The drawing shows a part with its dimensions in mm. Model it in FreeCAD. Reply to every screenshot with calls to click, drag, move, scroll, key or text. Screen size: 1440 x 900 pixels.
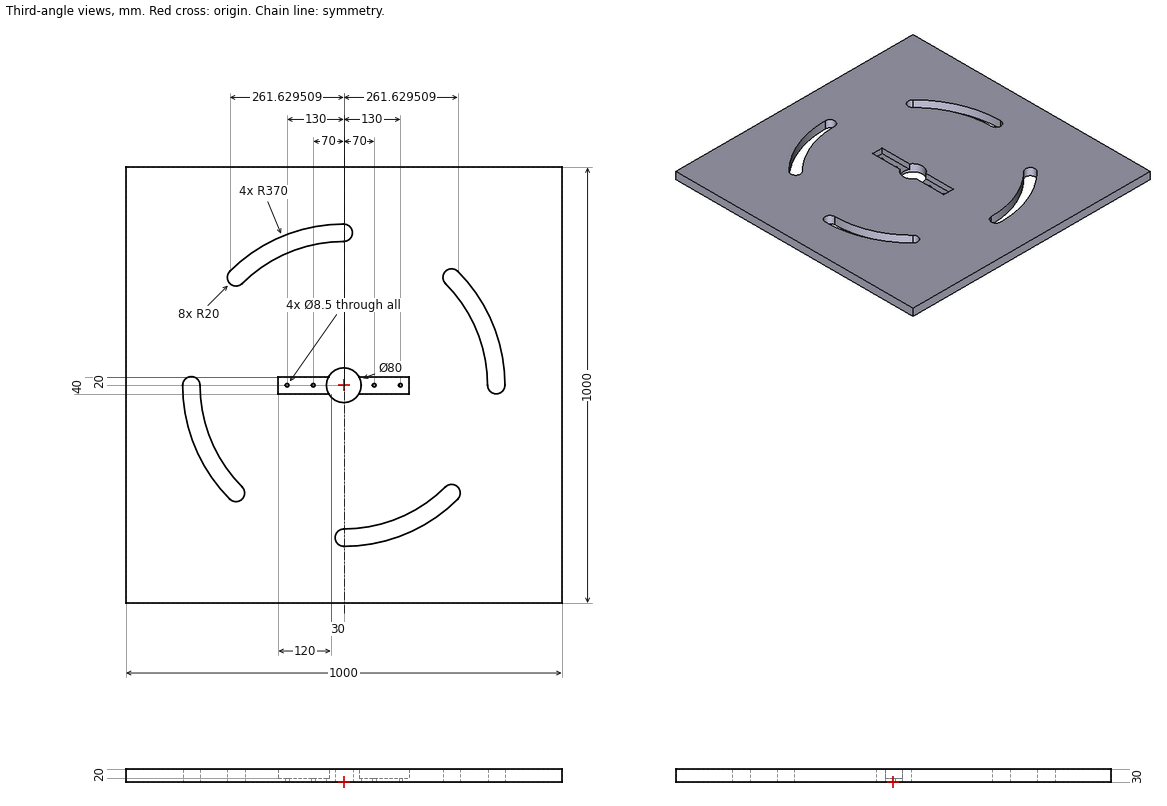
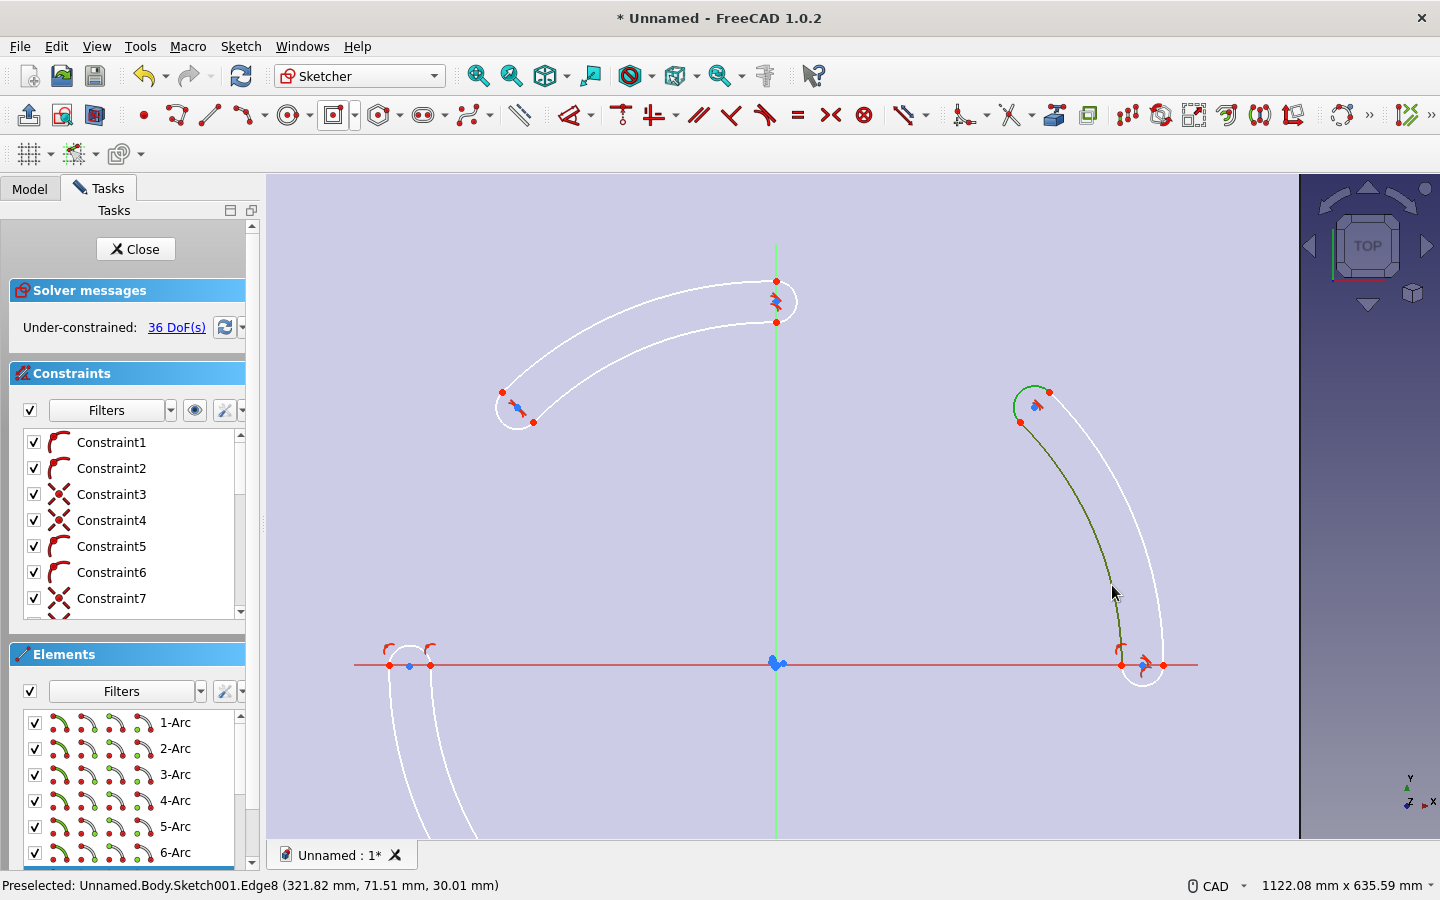
key(t)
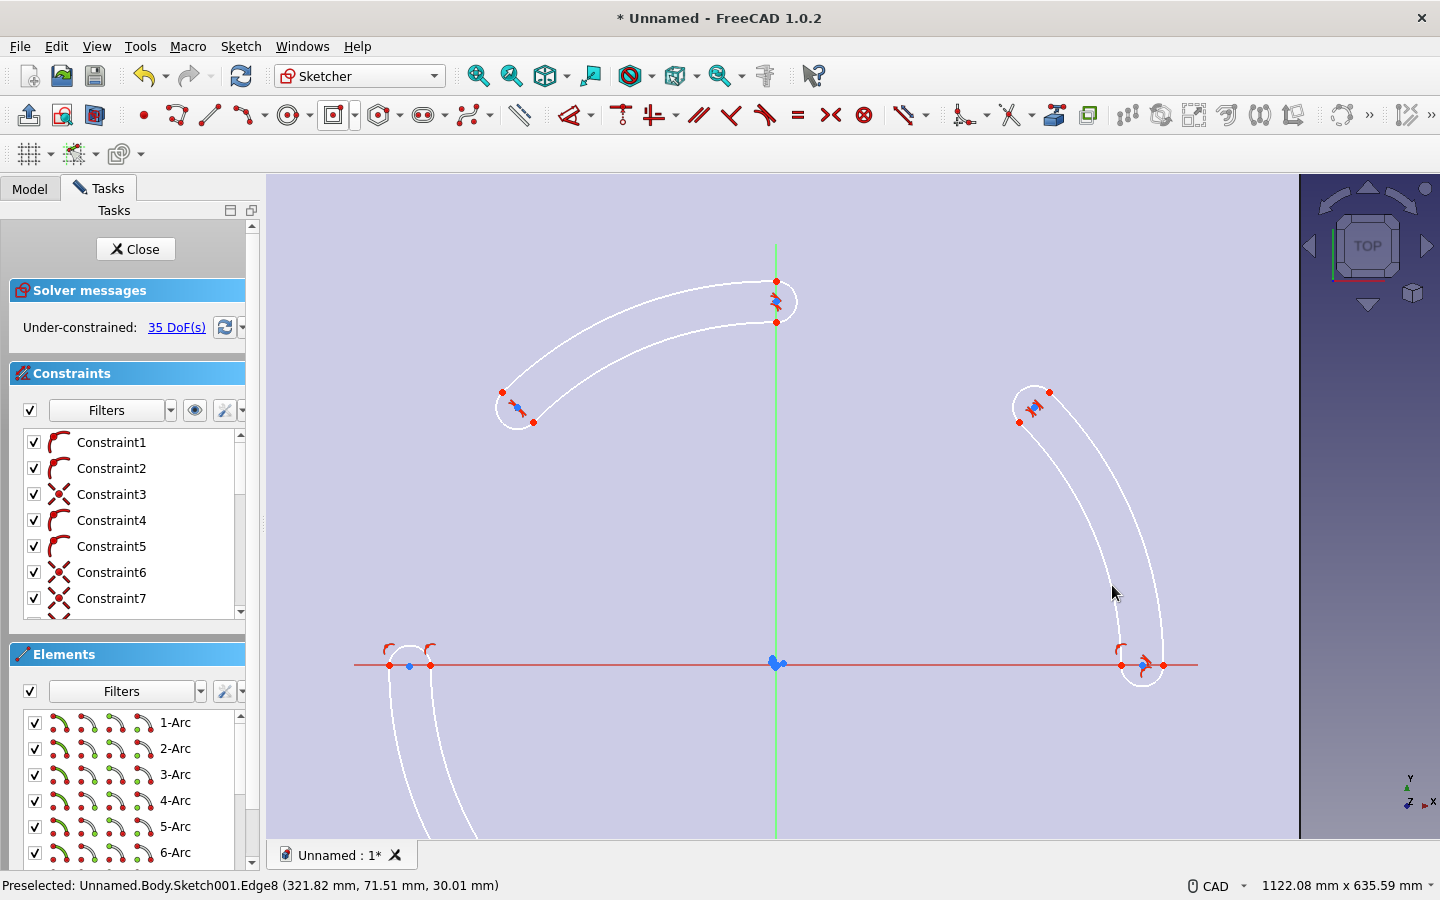
scroll(794, 313, down, 3)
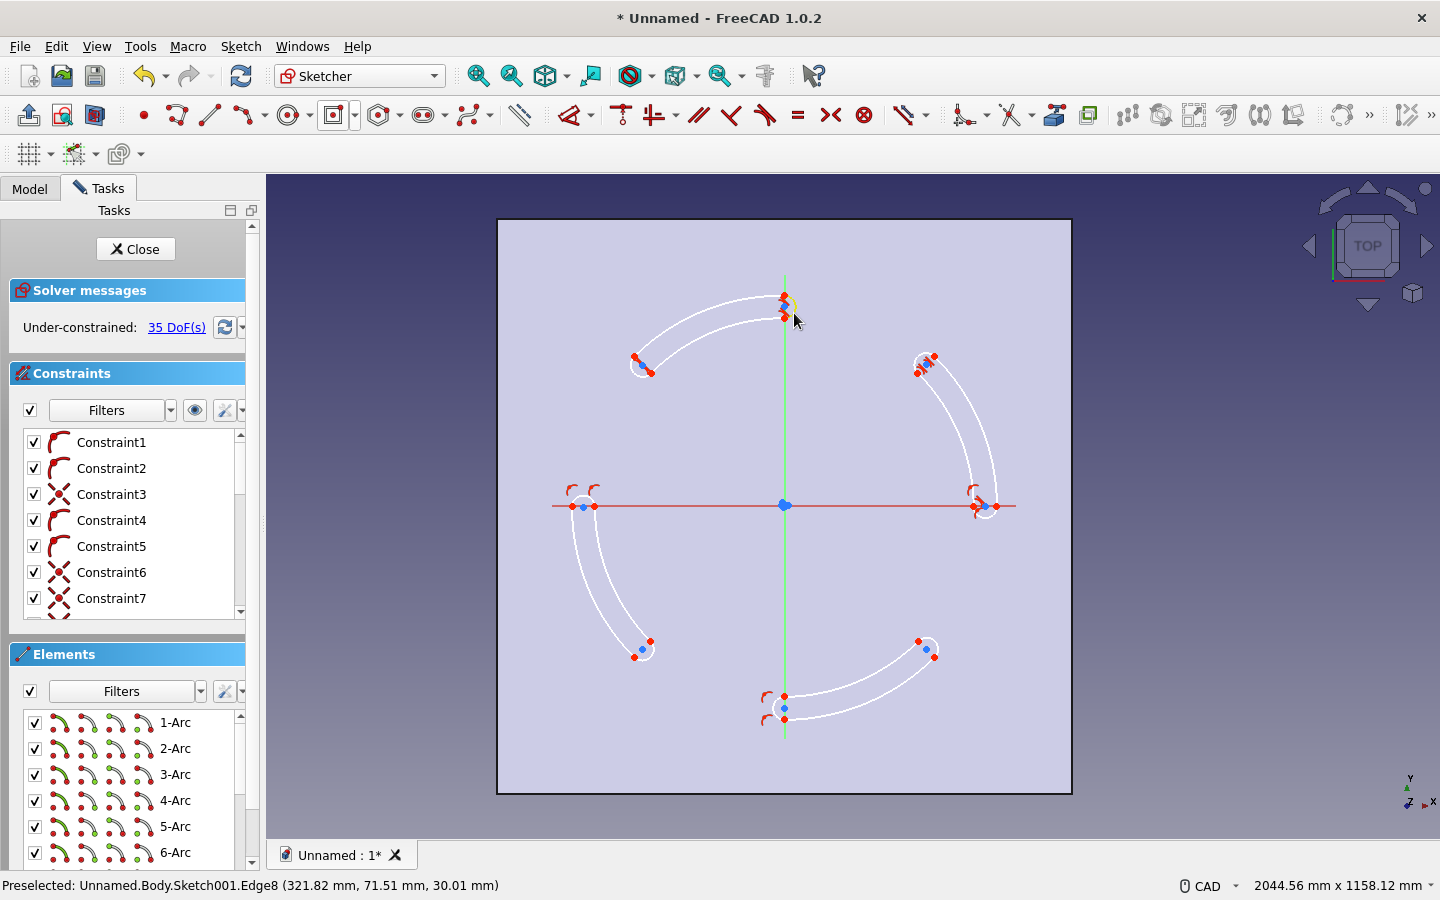
scroll(775, 702, up, 3)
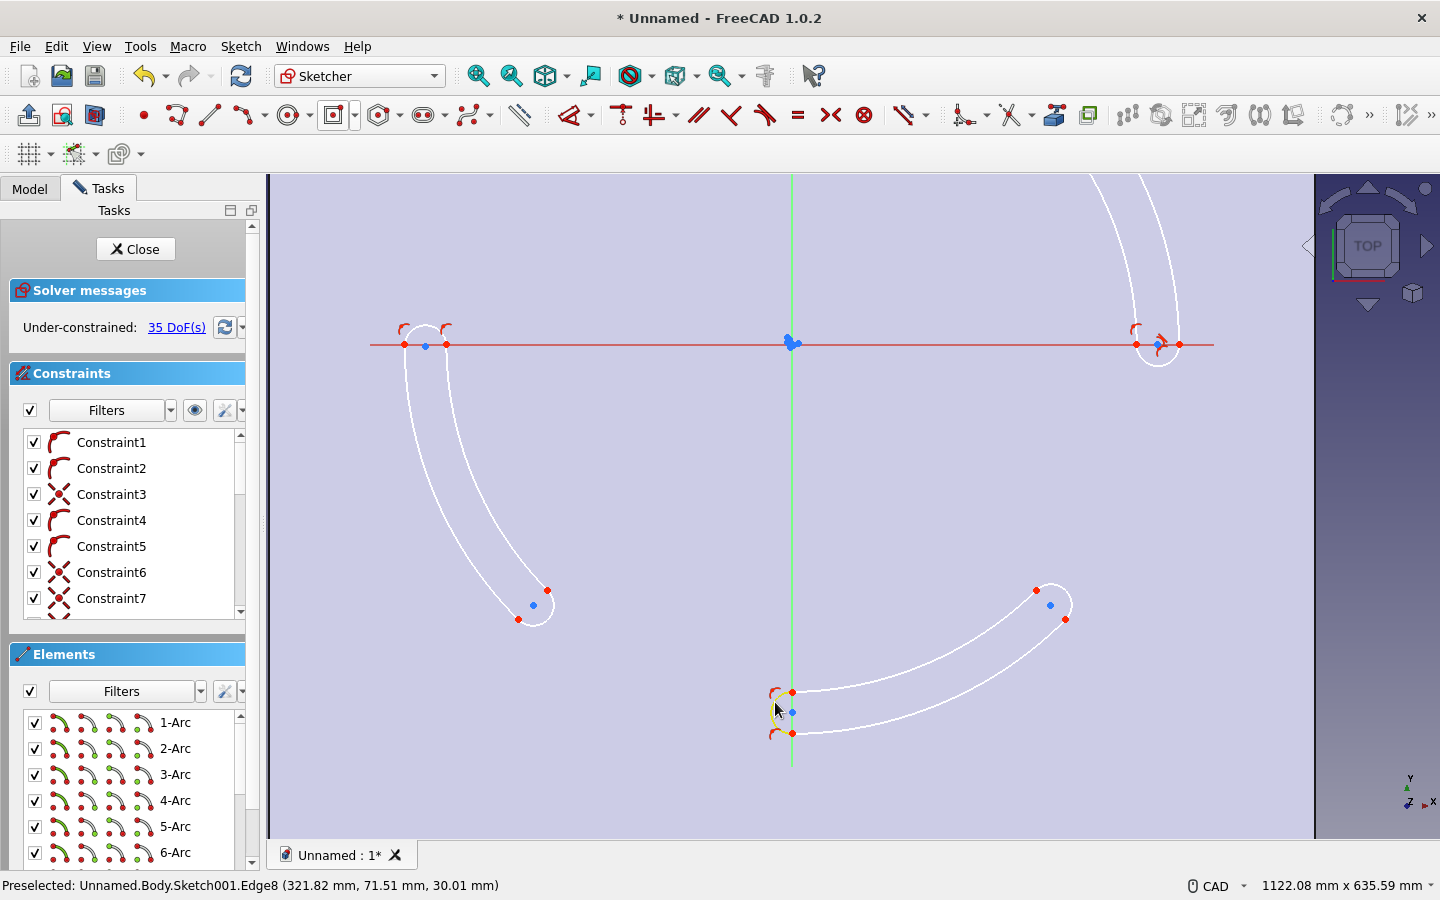
click(775, 701)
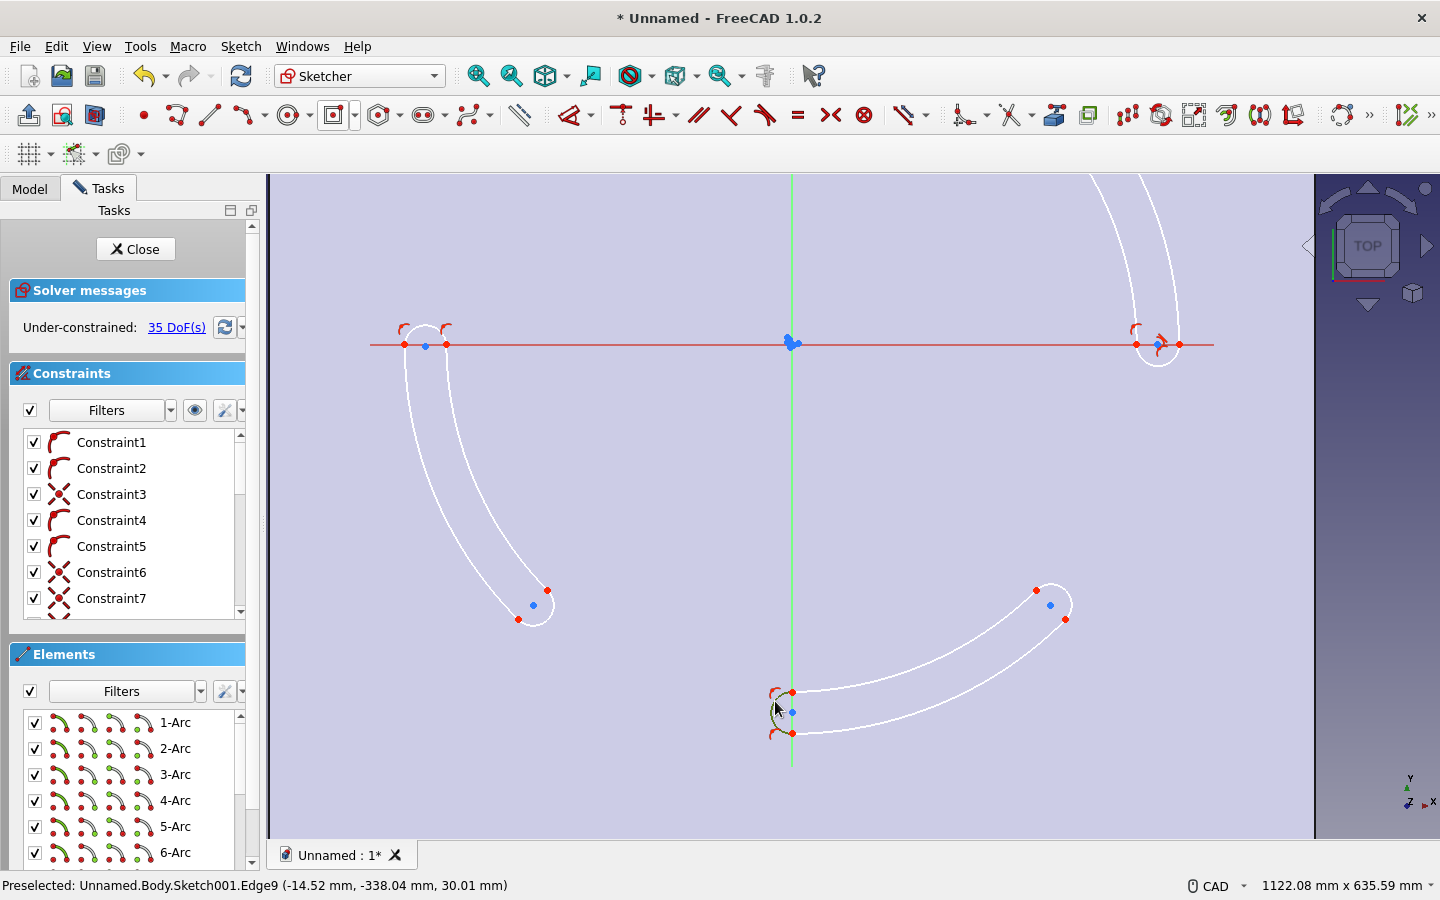
click(882, 723)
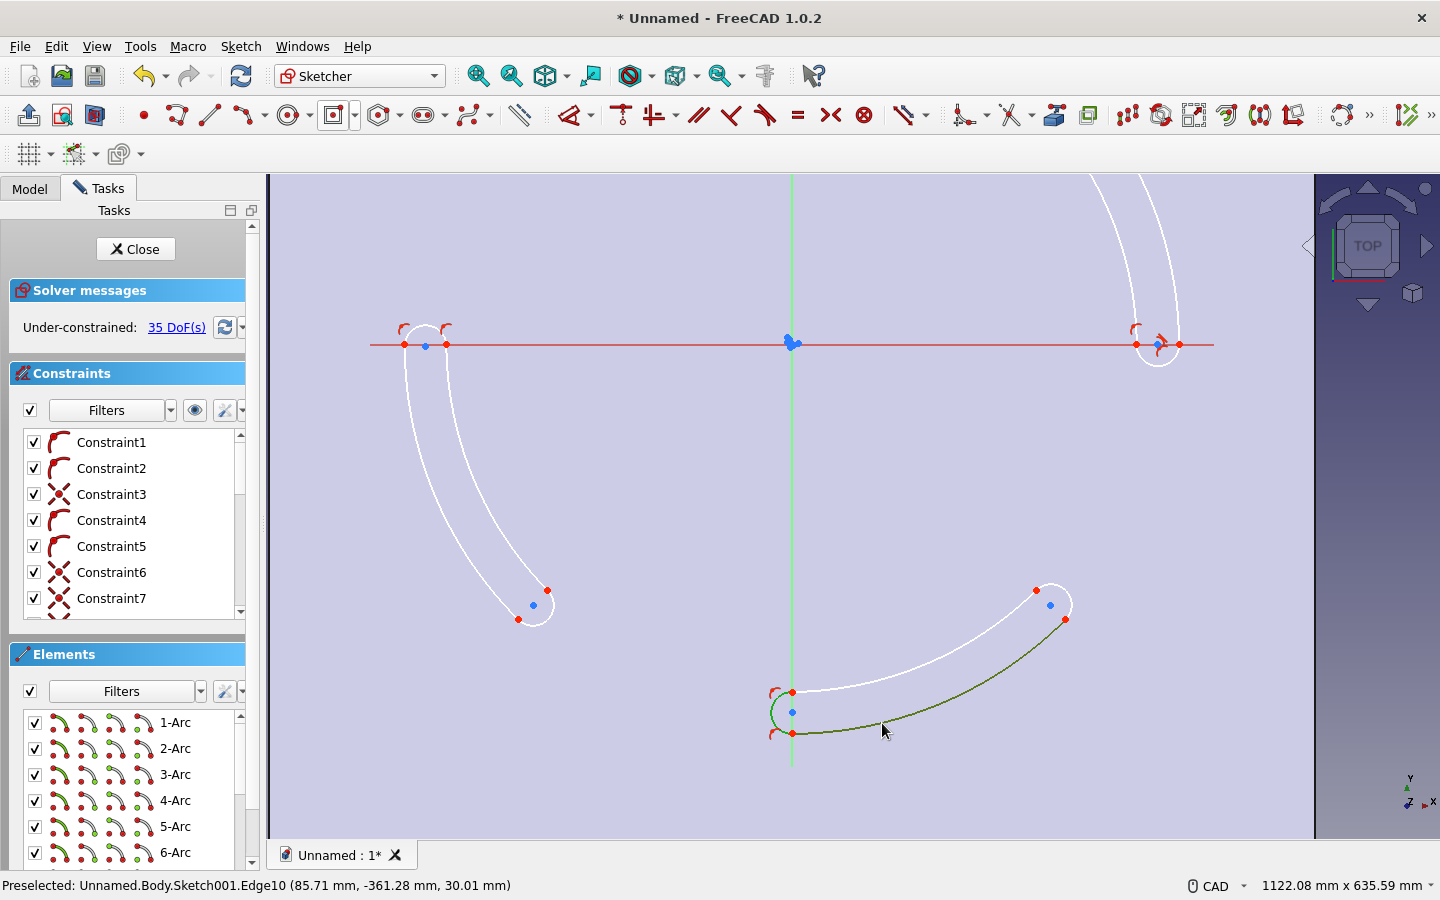
click(765, 116)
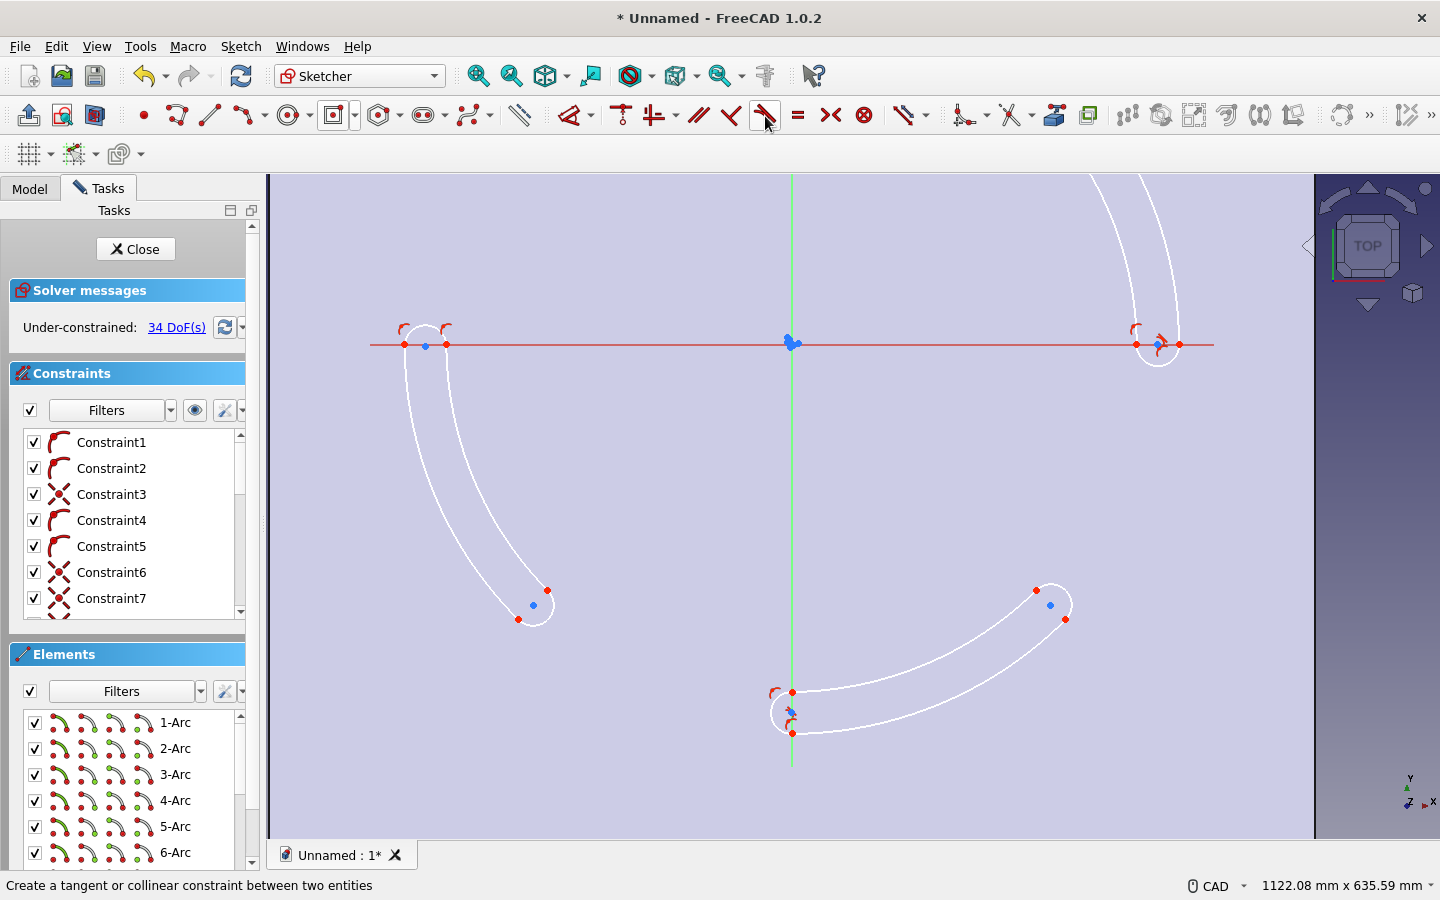
click(882, 723)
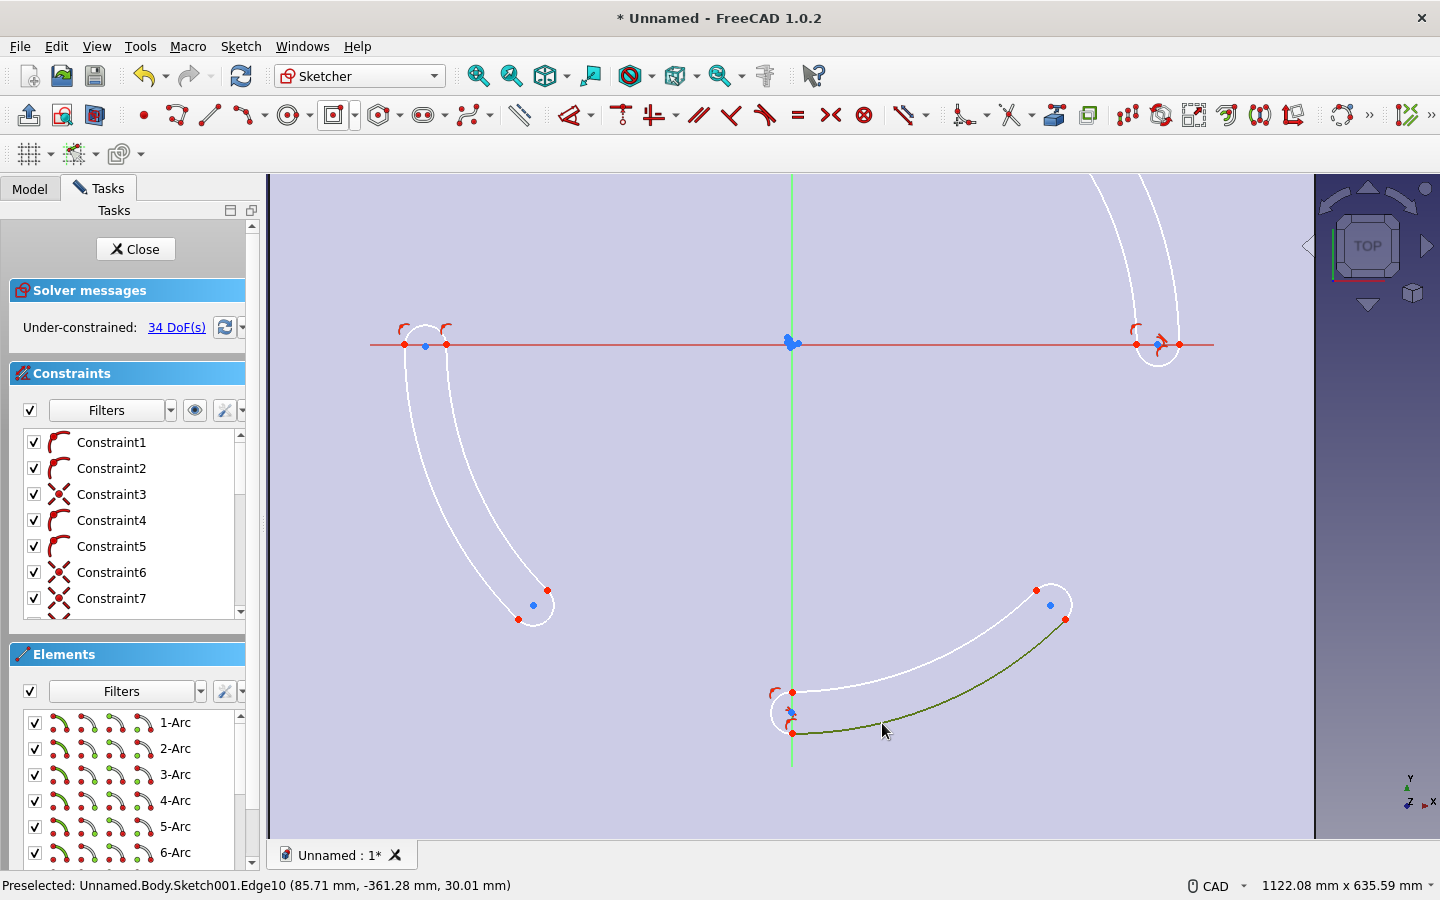
click(1071, 602)